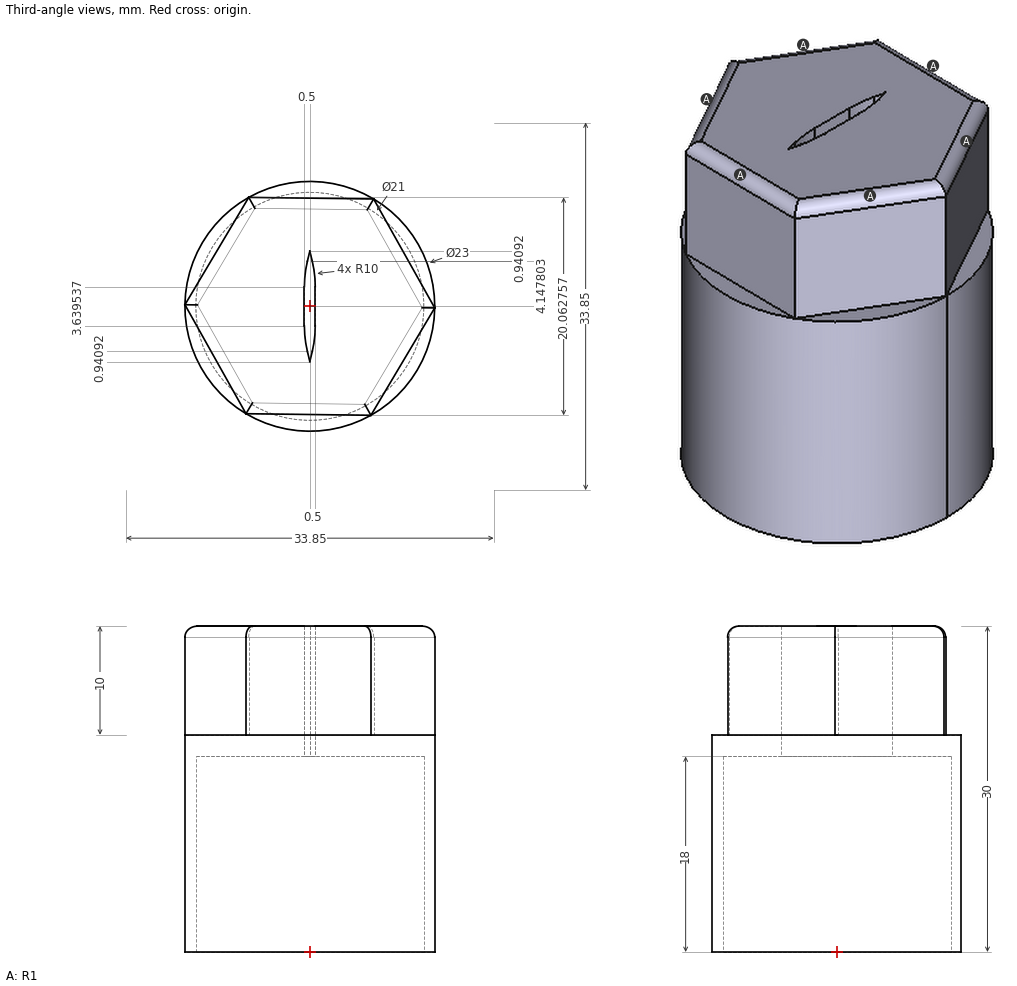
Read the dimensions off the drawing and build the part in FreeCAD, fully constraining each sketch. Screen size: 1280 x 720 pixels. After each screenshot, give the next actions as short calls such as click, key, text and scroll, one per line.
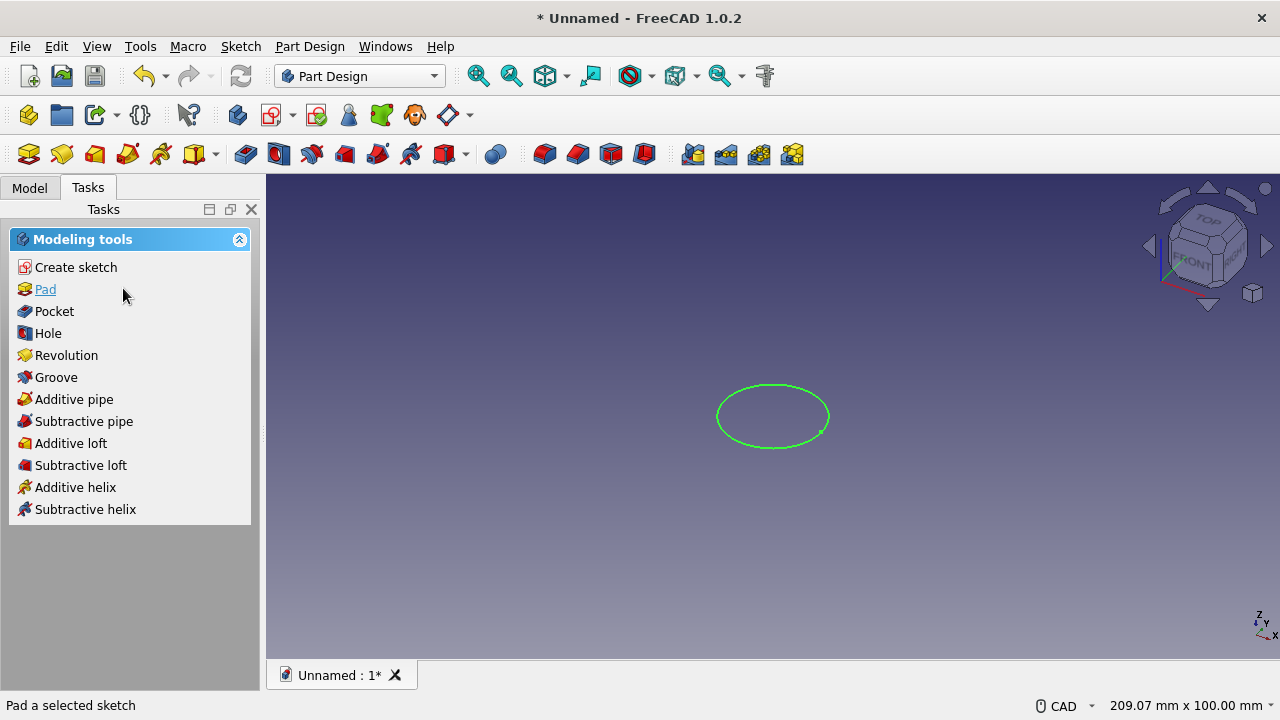
click(29, 154)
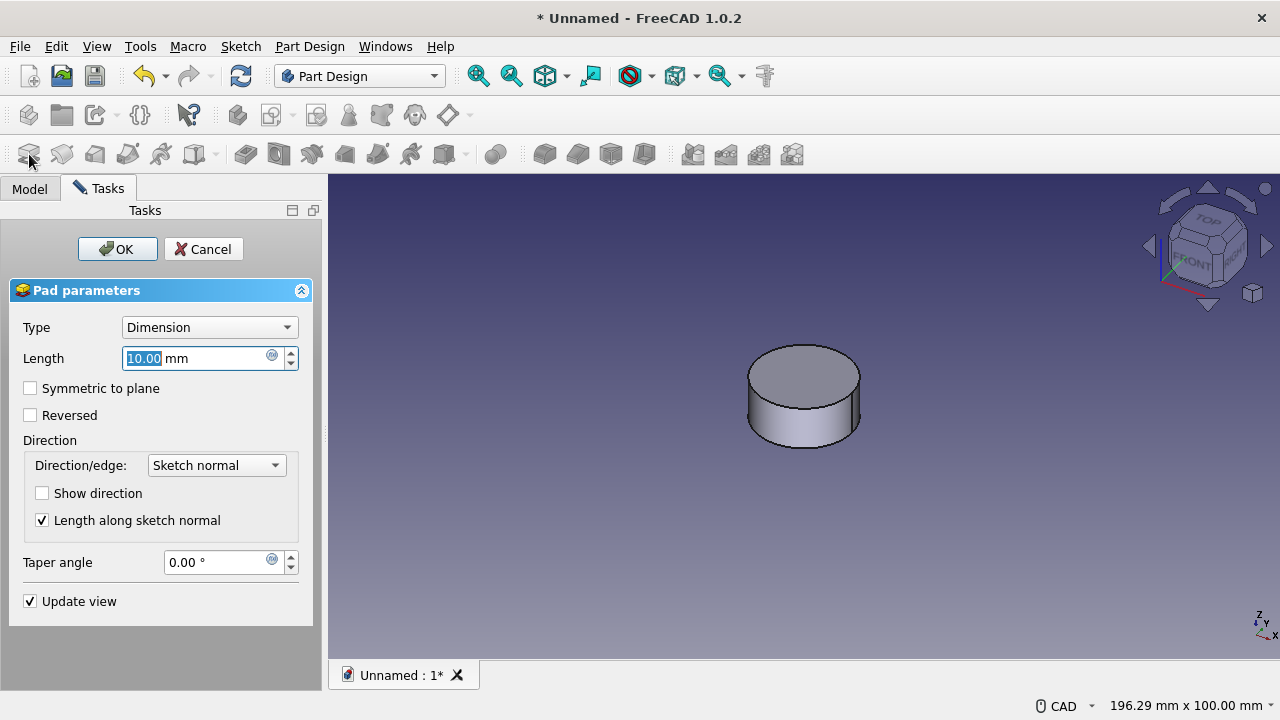
text(30)
key(Tab)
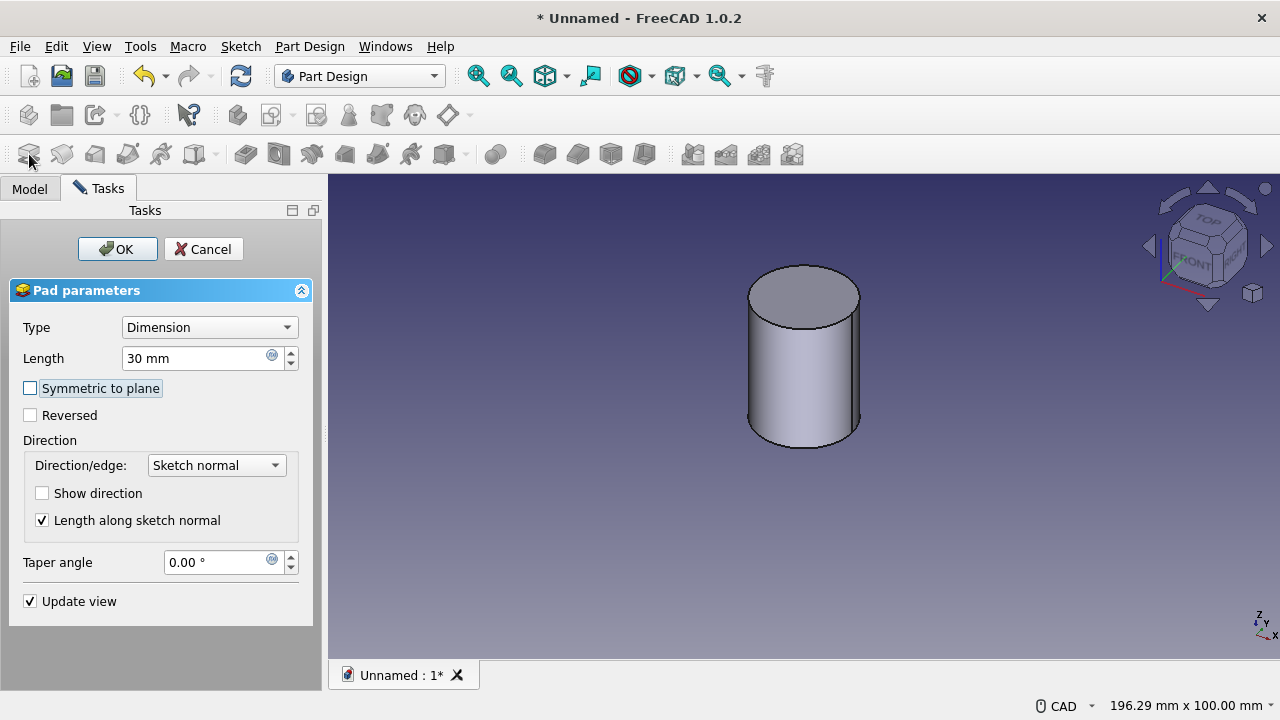
click(118, 249)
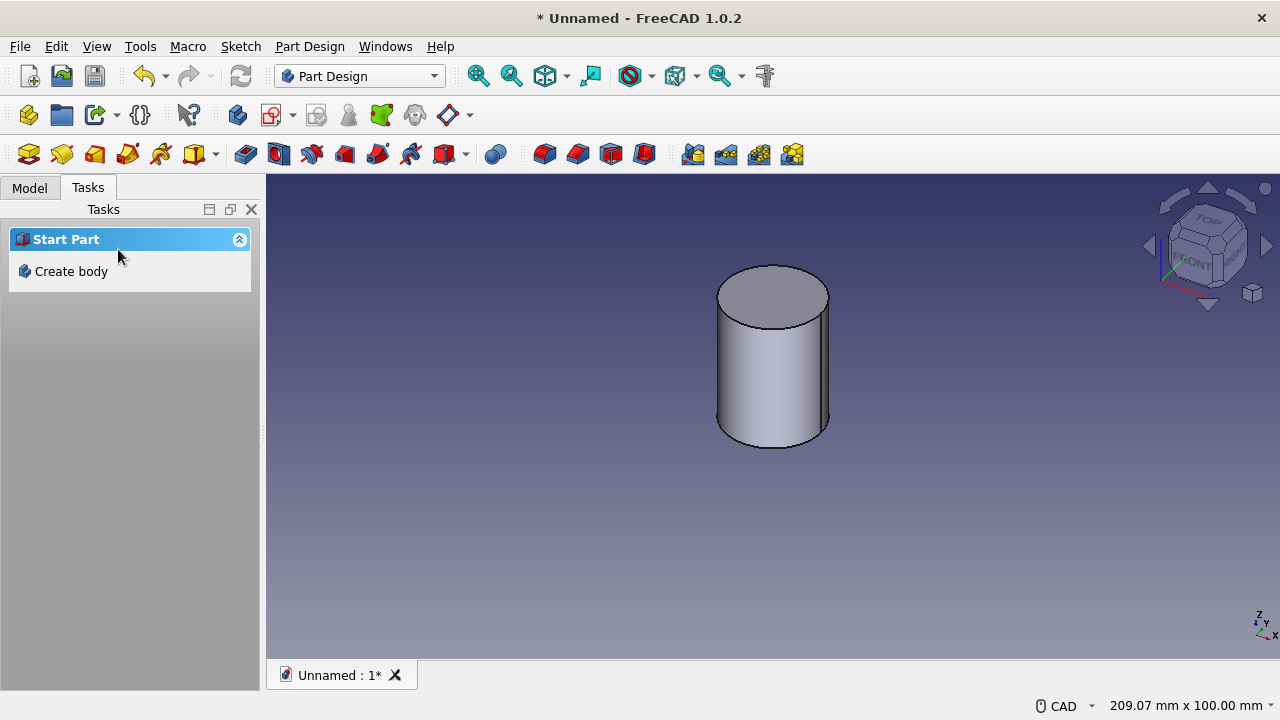
click(479, 76)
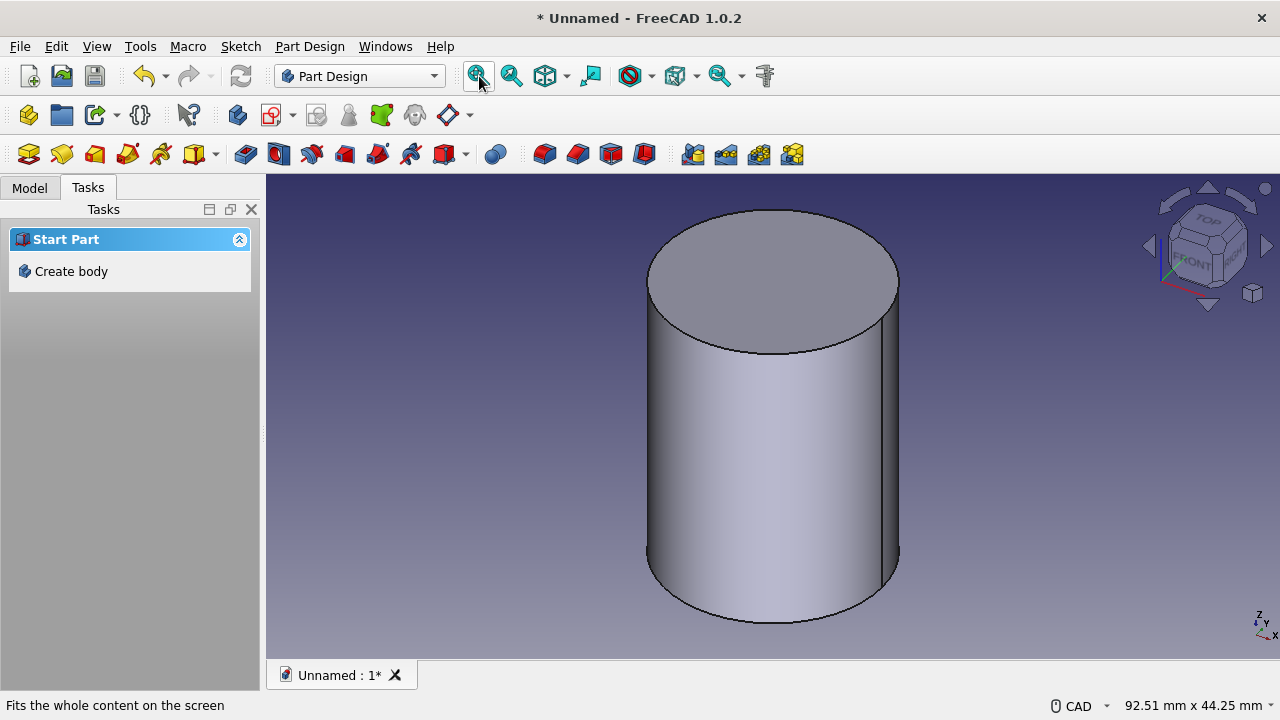
click(773, 281)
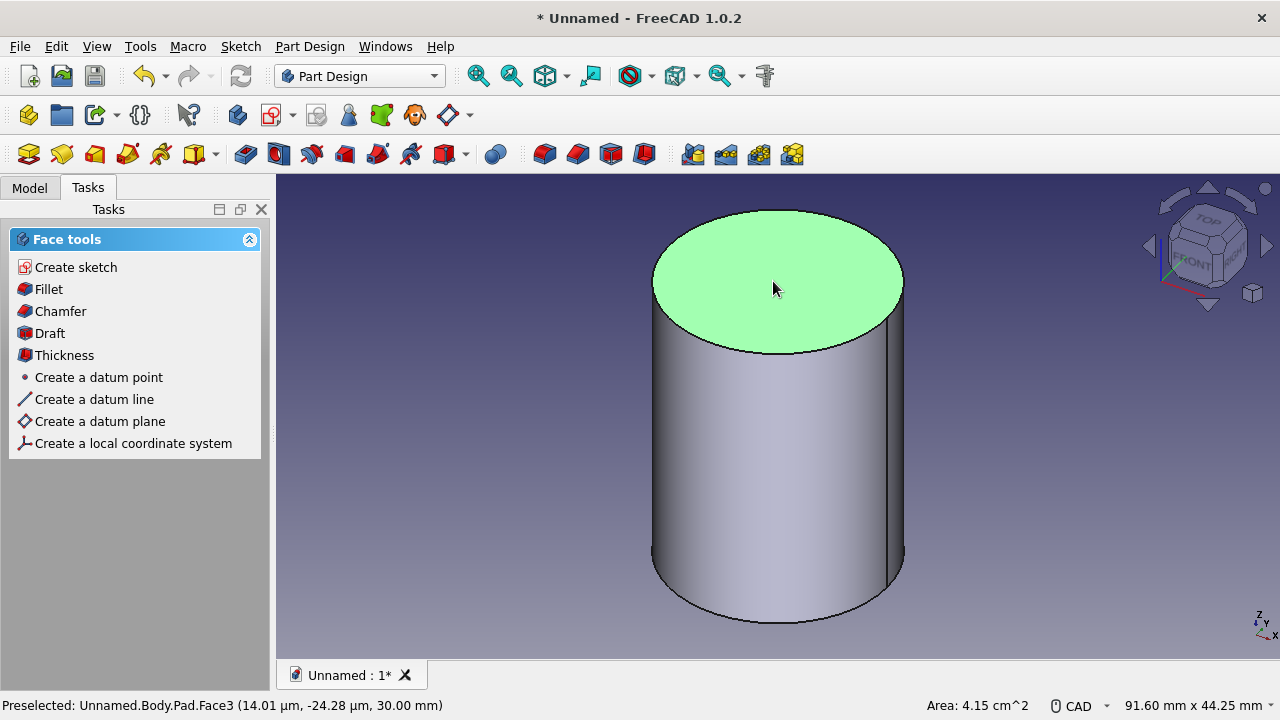
click(270, 116)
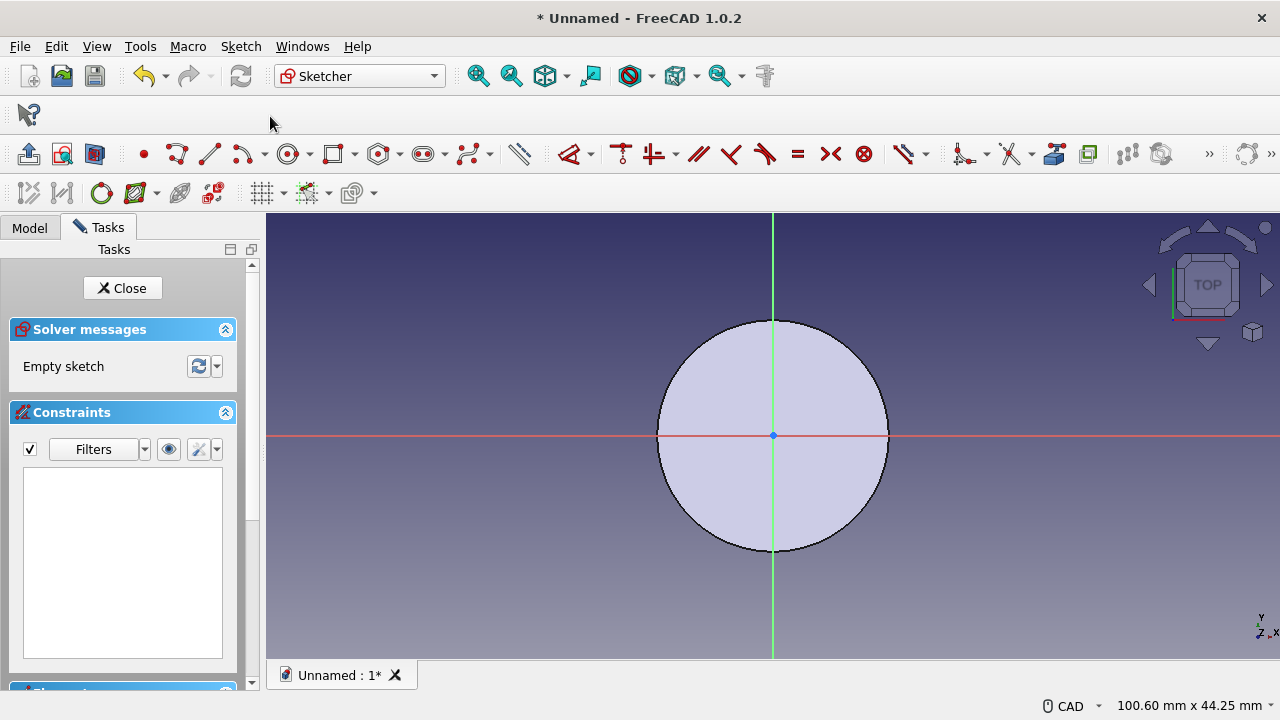
scroll(395, 436, down, 1)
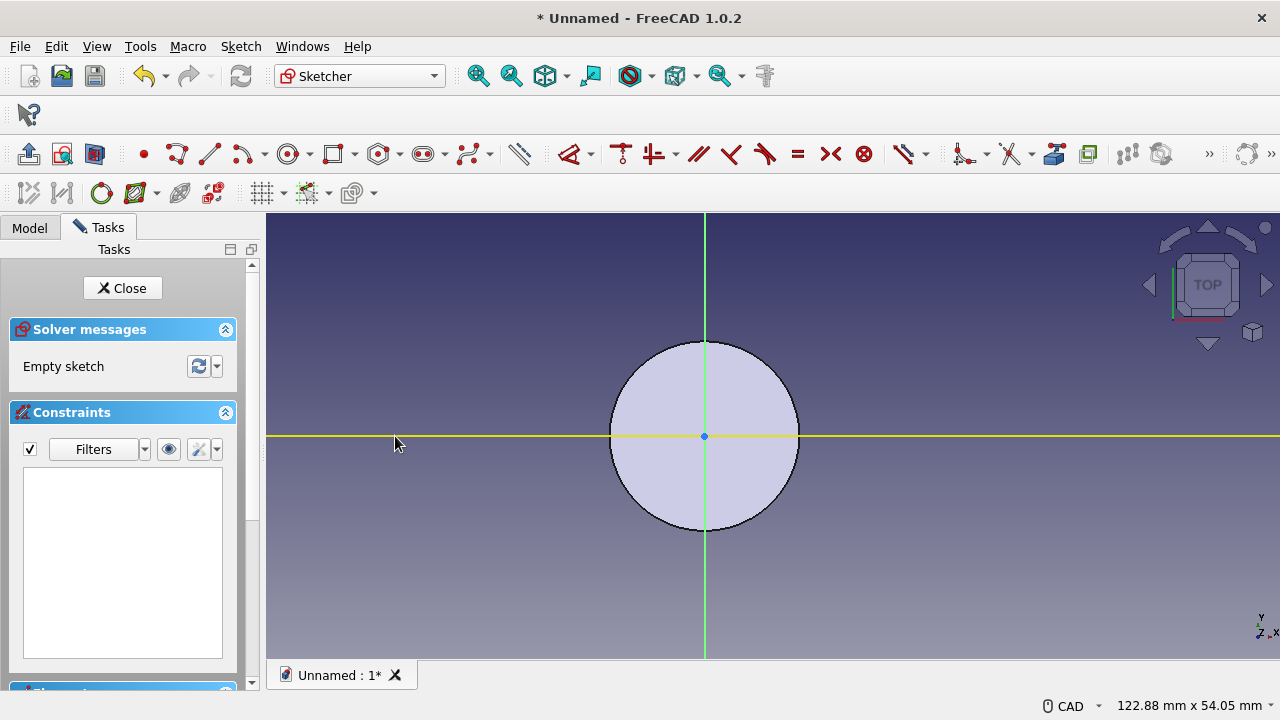
click(354, 154)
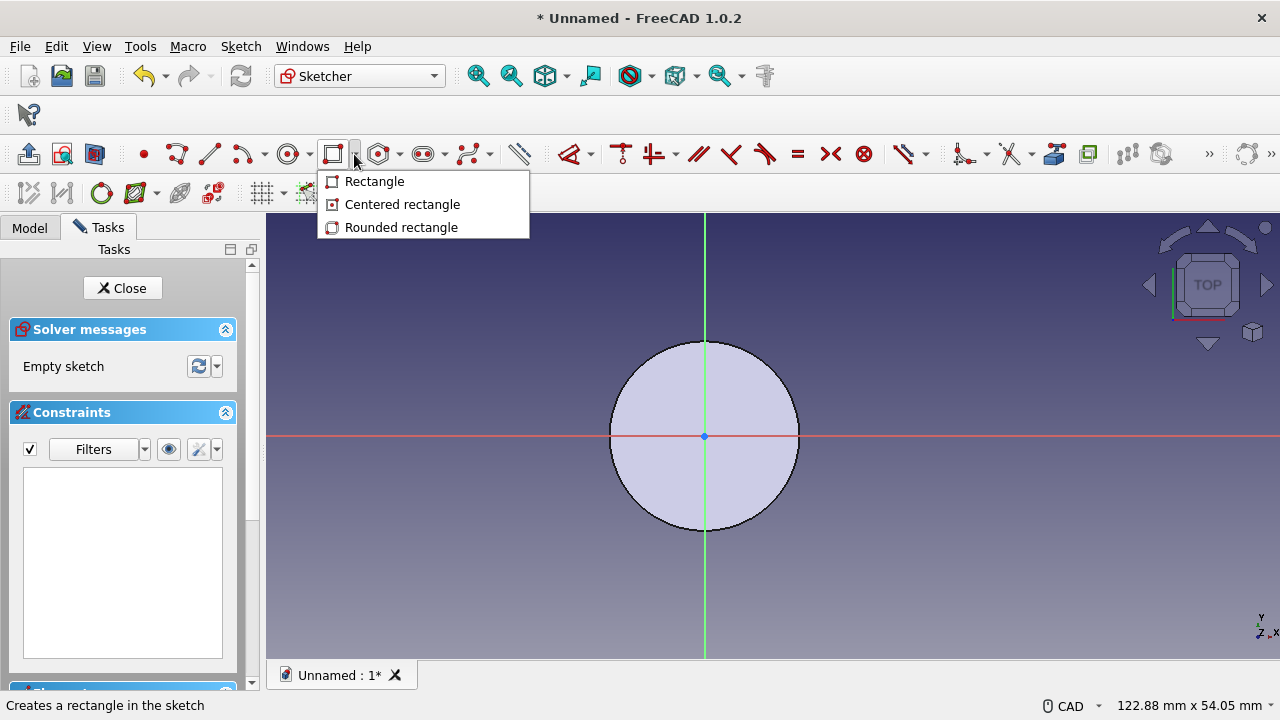
click(424, 204)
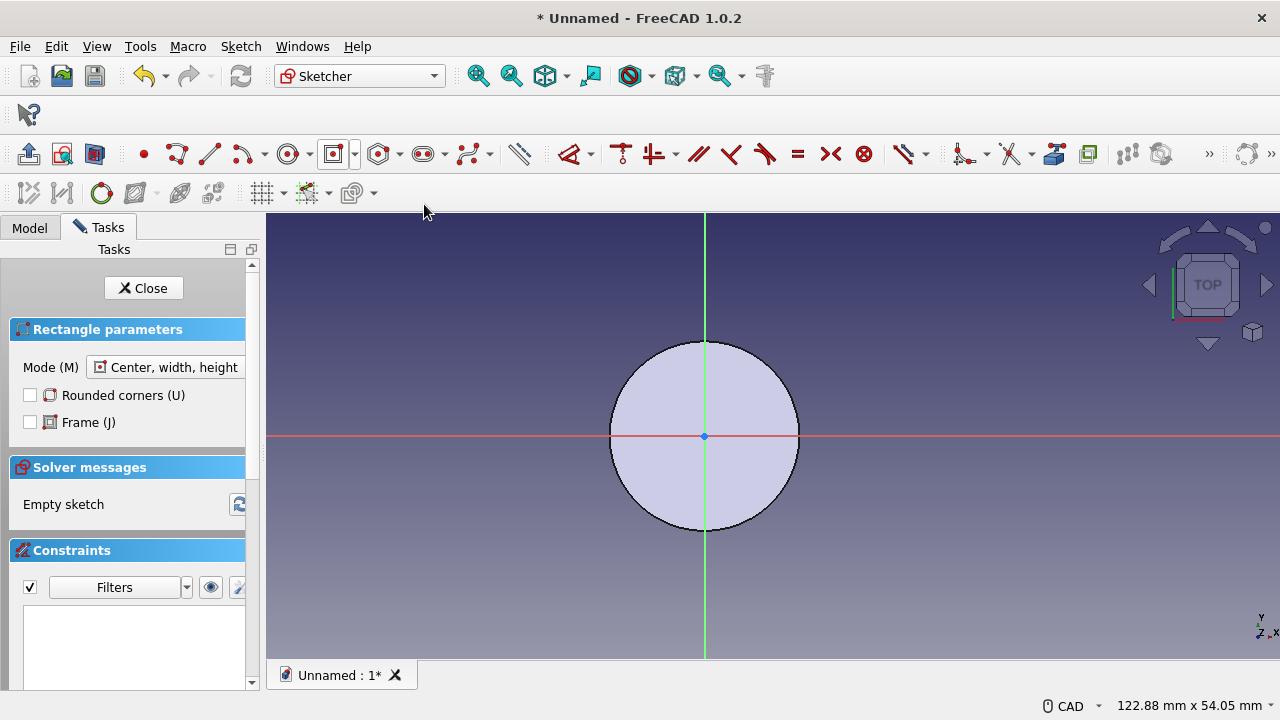
click(705, 436)
click(844, 296)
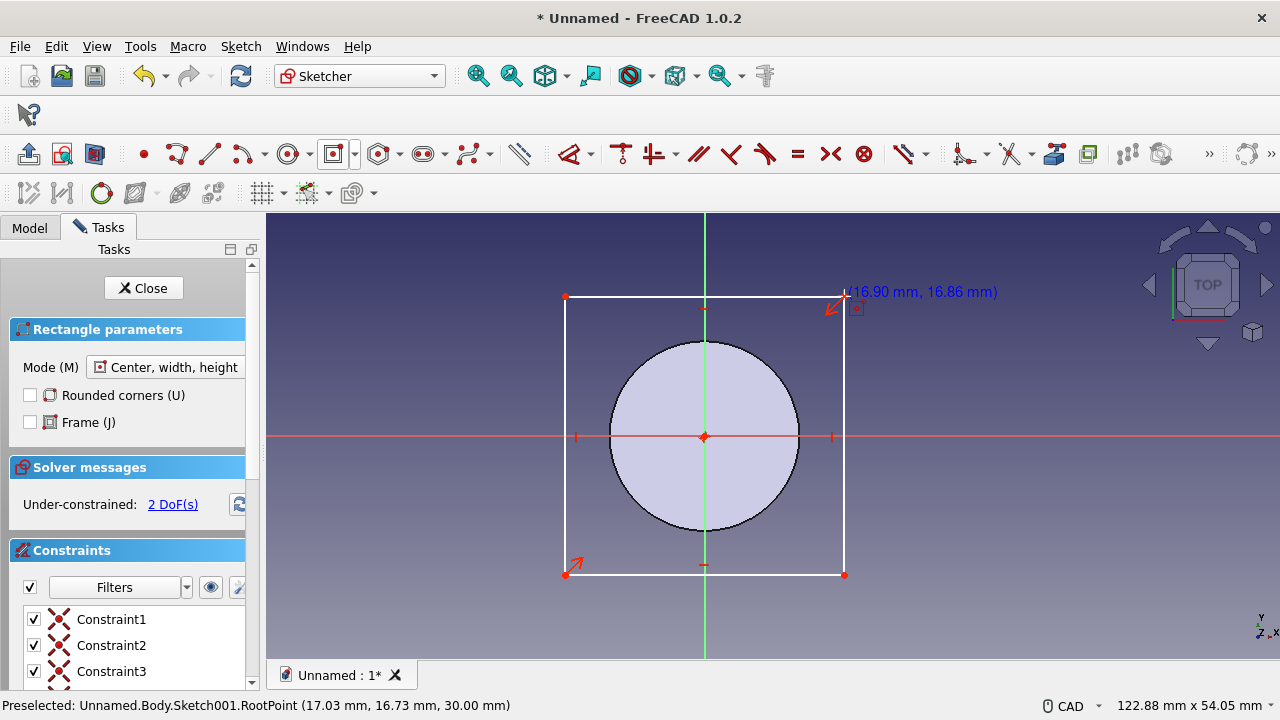
click(378, 154)